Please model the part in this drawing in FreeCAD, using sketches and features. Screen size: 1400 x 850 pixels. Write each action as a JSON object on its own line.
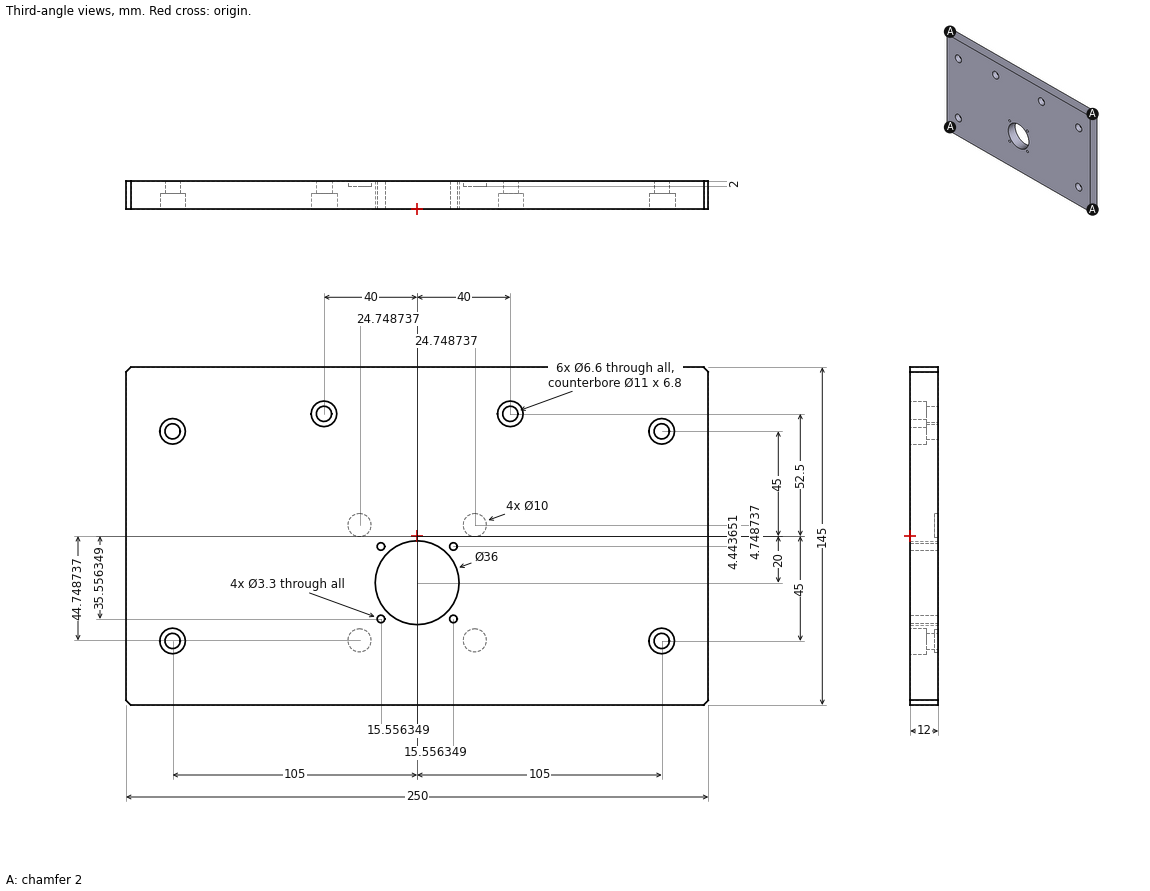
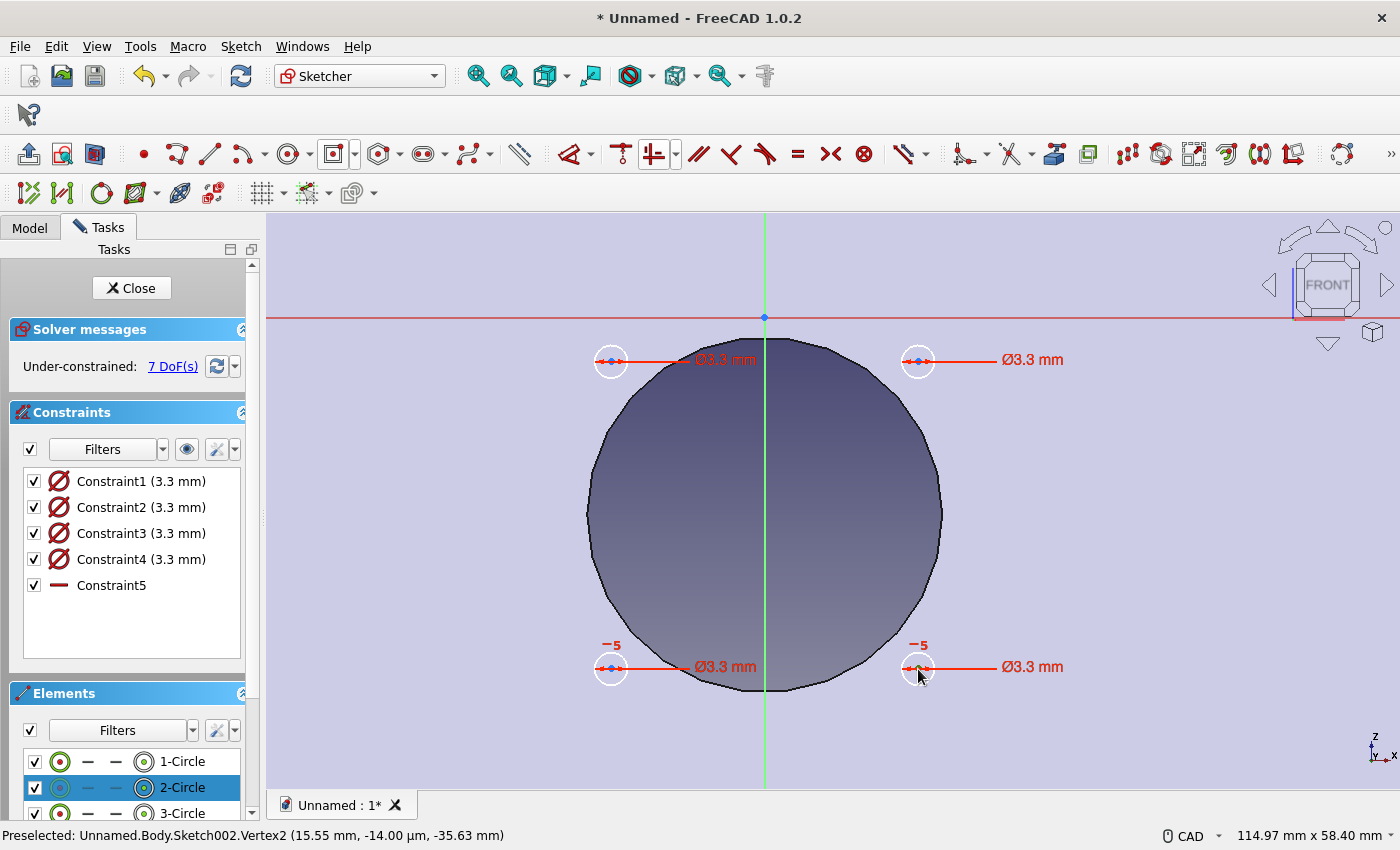
{"action": "left_click", "coordinate": [918, 362]}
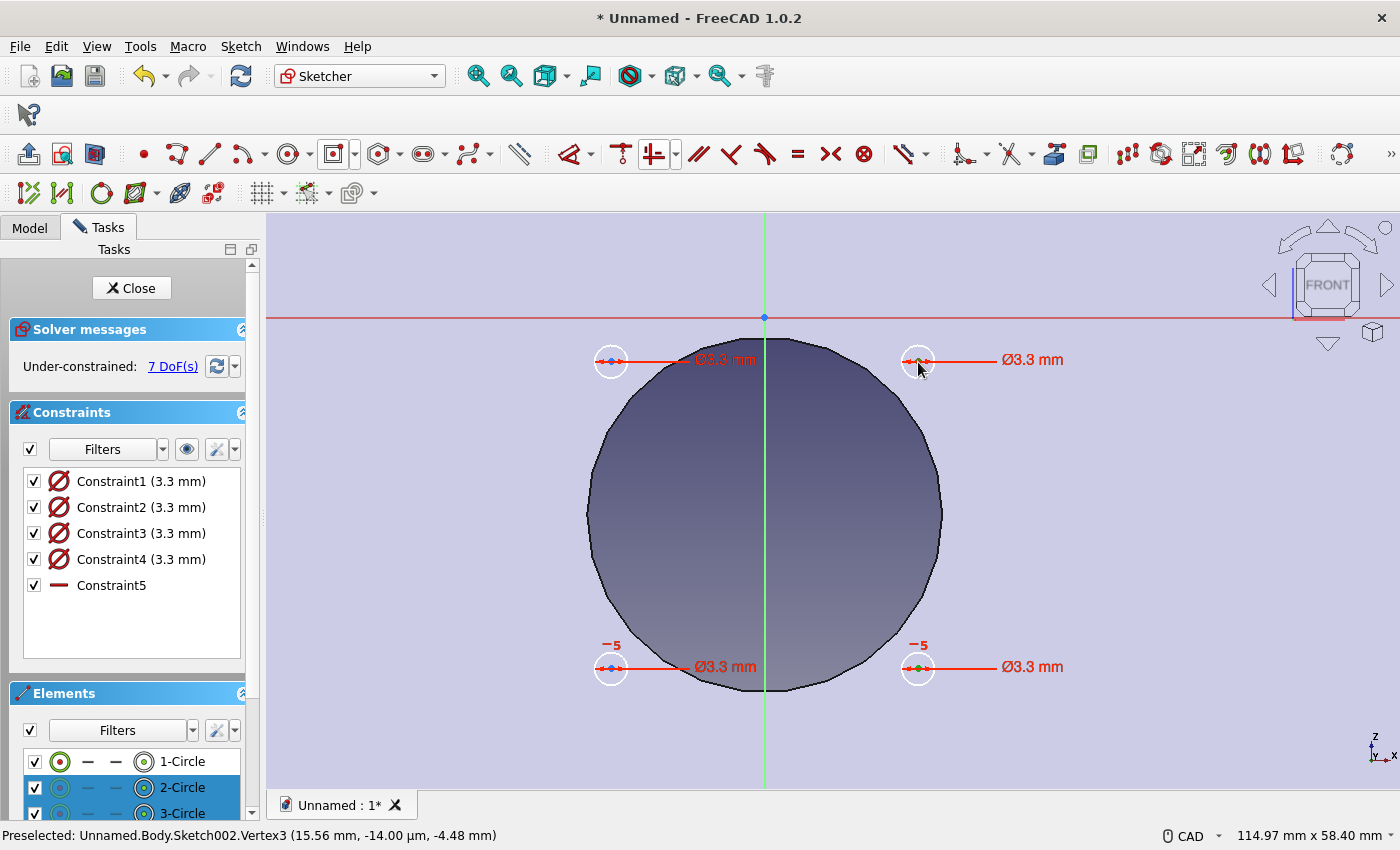
{"action": "key", "text": "v"}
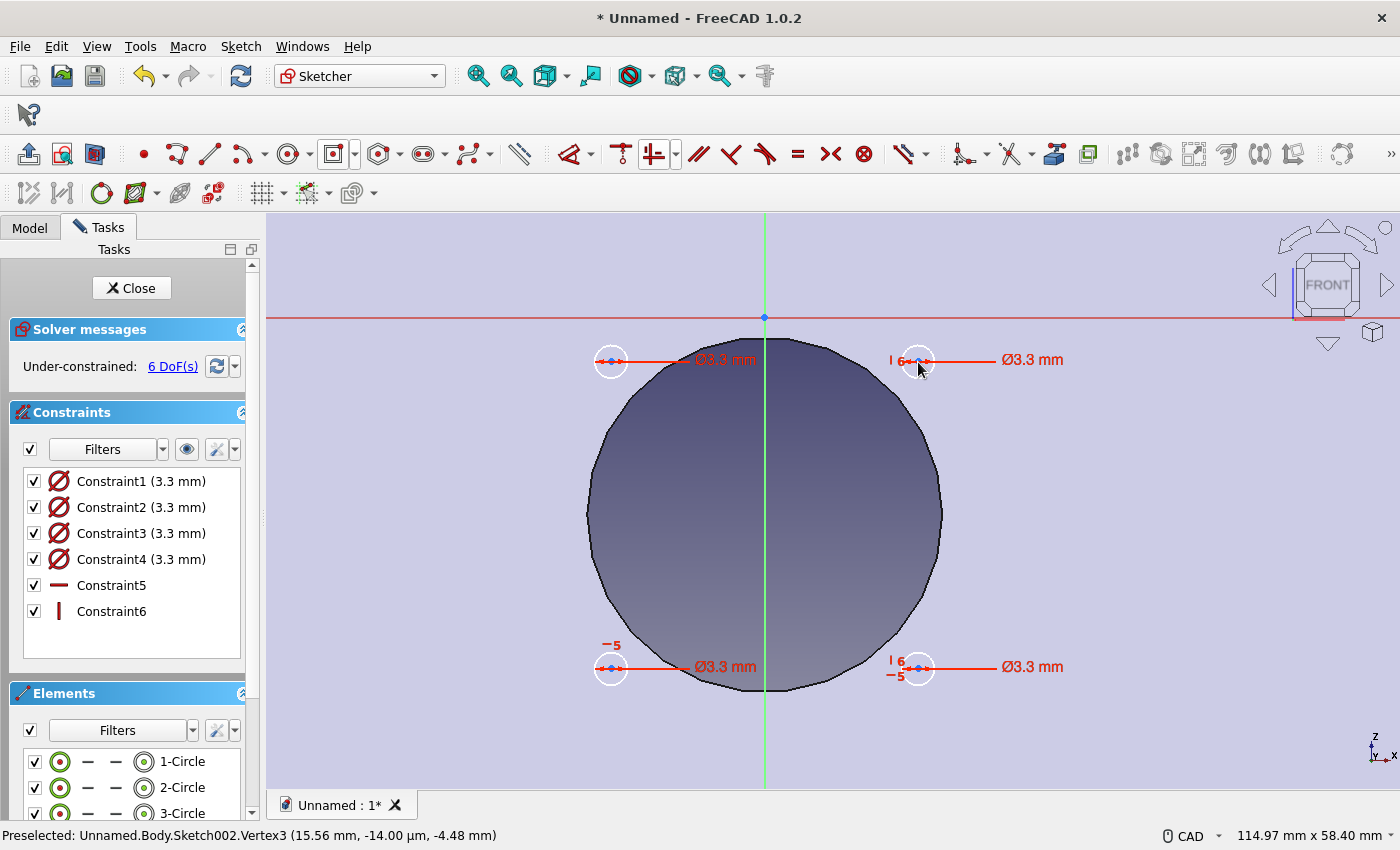
{"action": "left_click", "coordinate": [611, 669]}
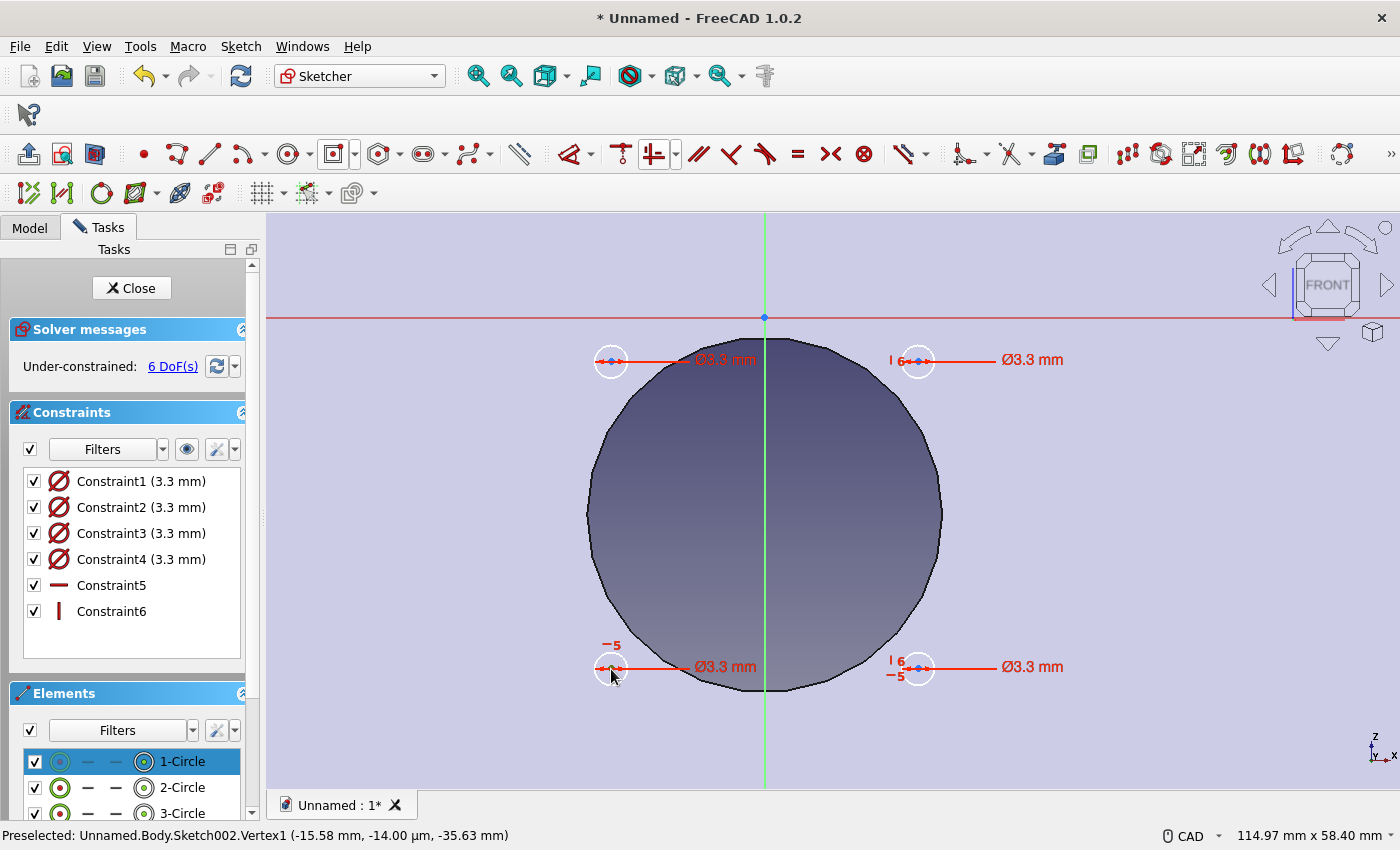
{"action": "left_click", "coordinate": [611, 362]}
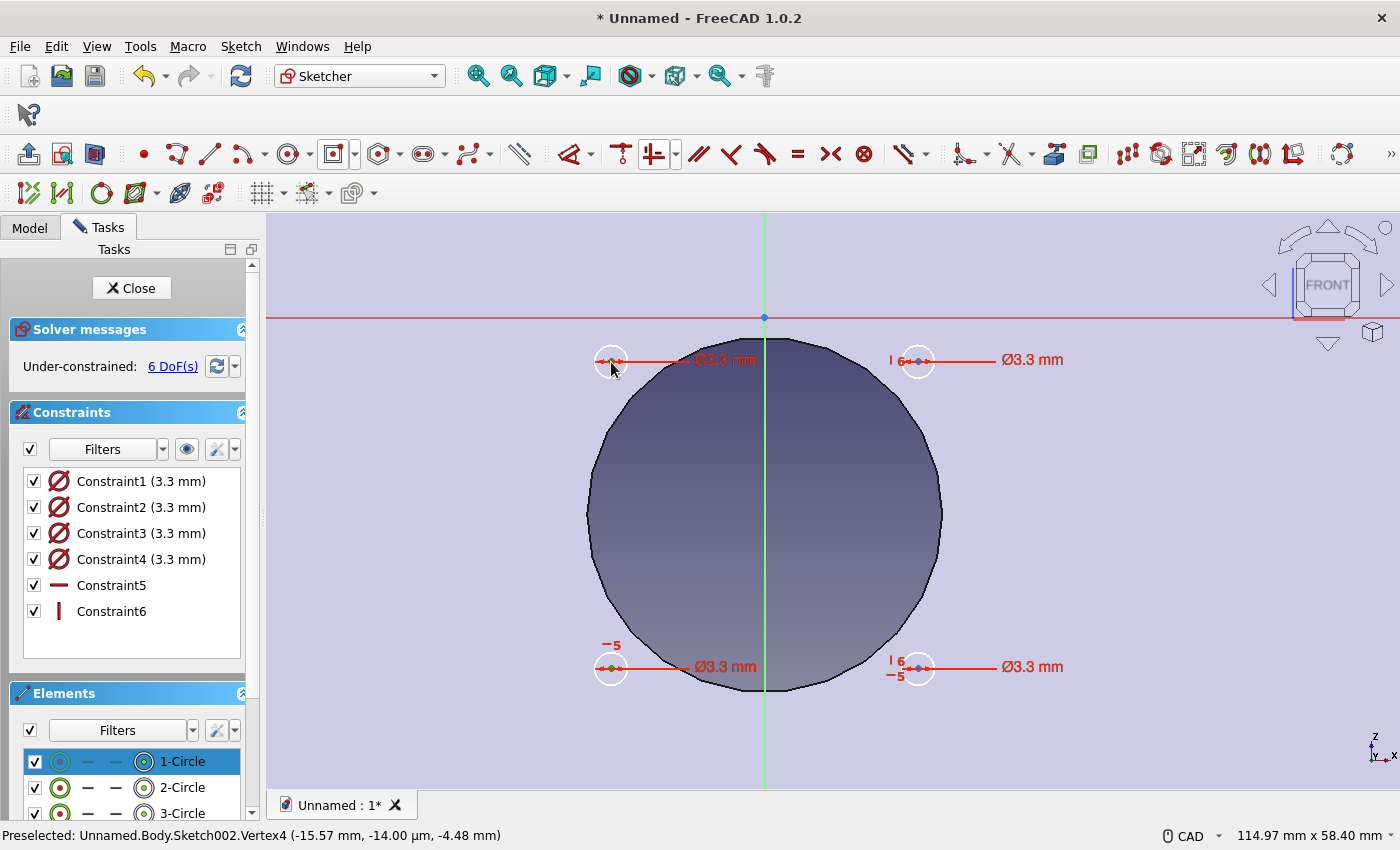
{"action": "left_click", "coordinate": [676, 154]}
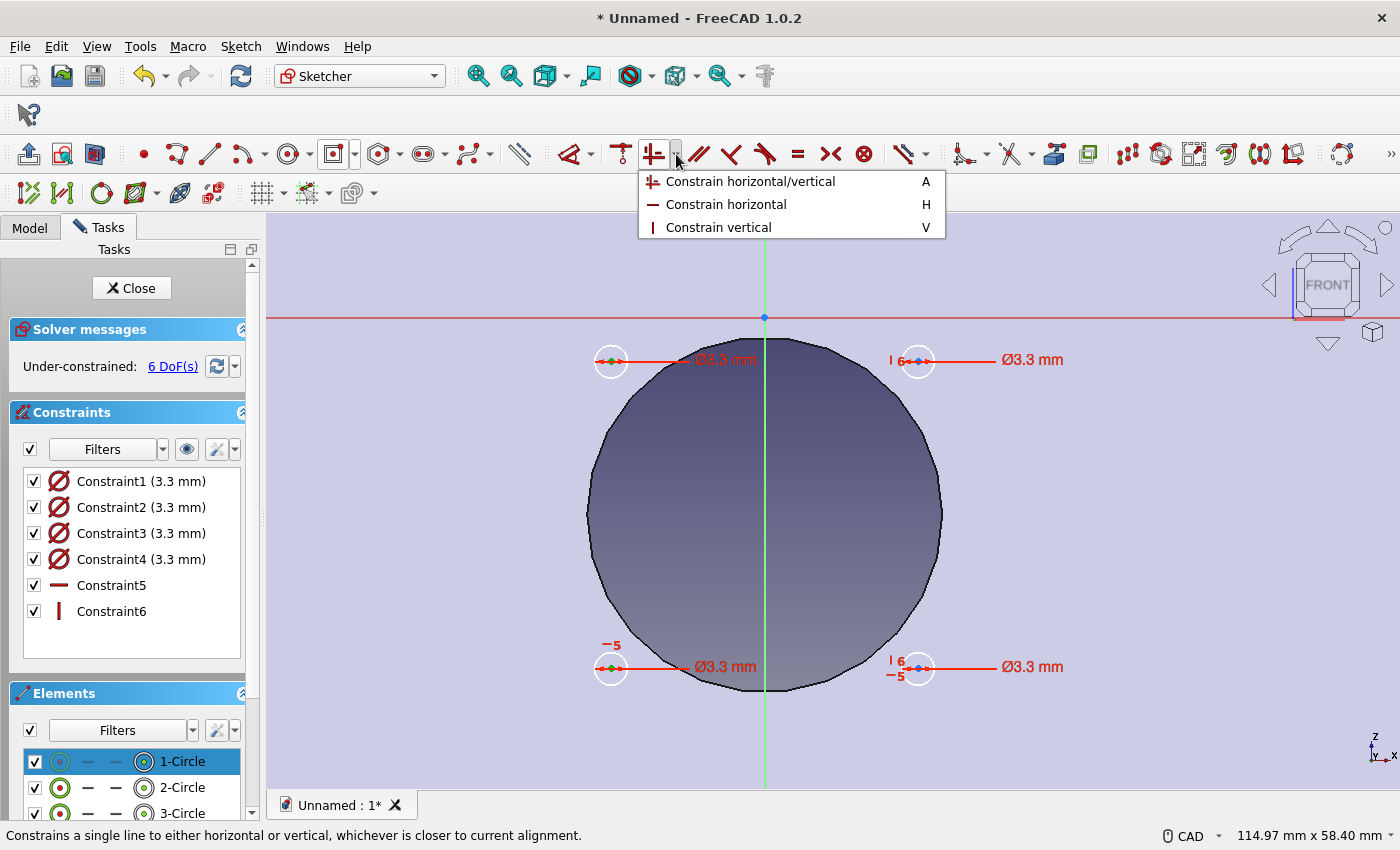
{"action": "left_click", "coordinate": [792, 228]}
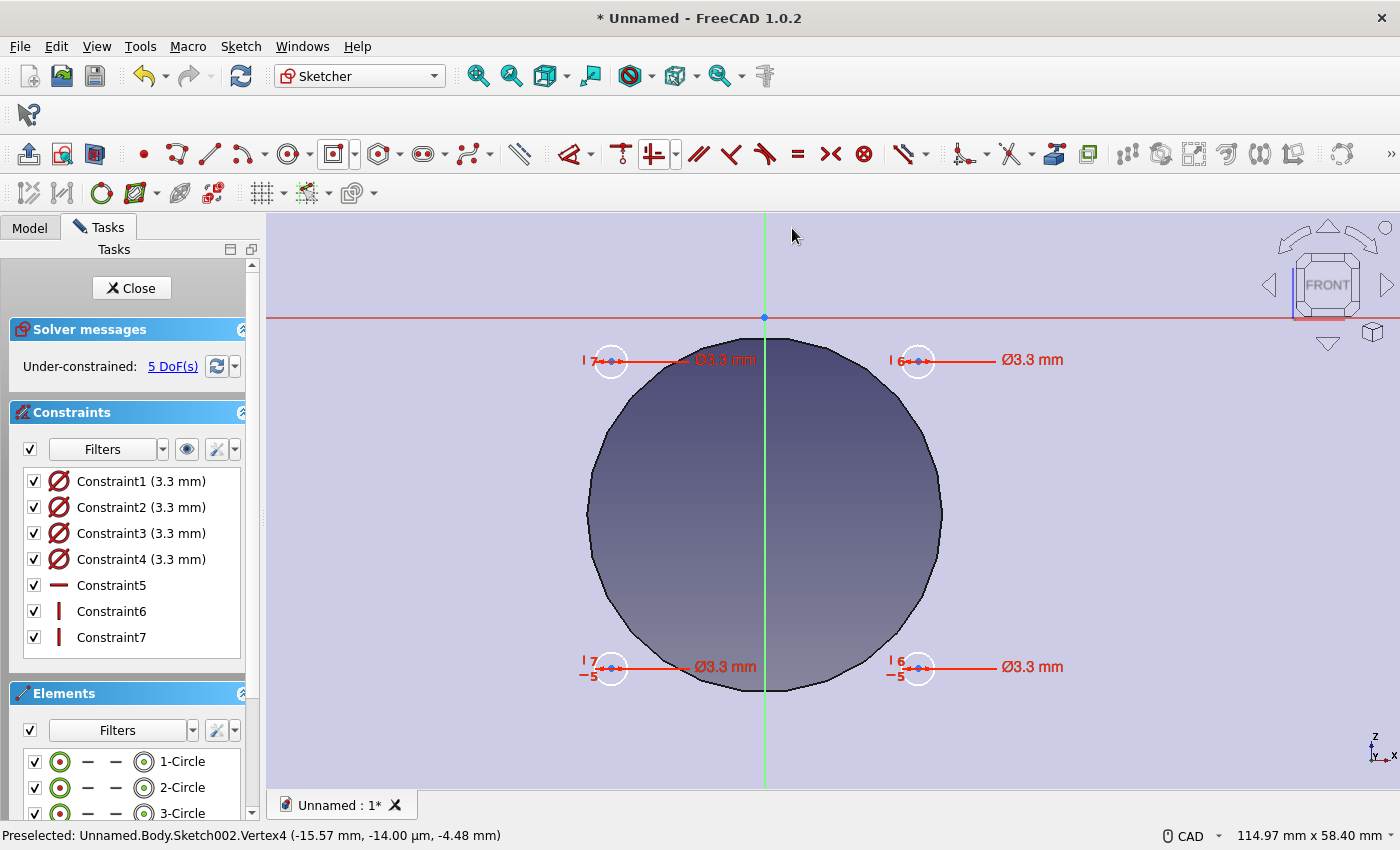
{"action": "left_click", "coordinate": [918, 362]}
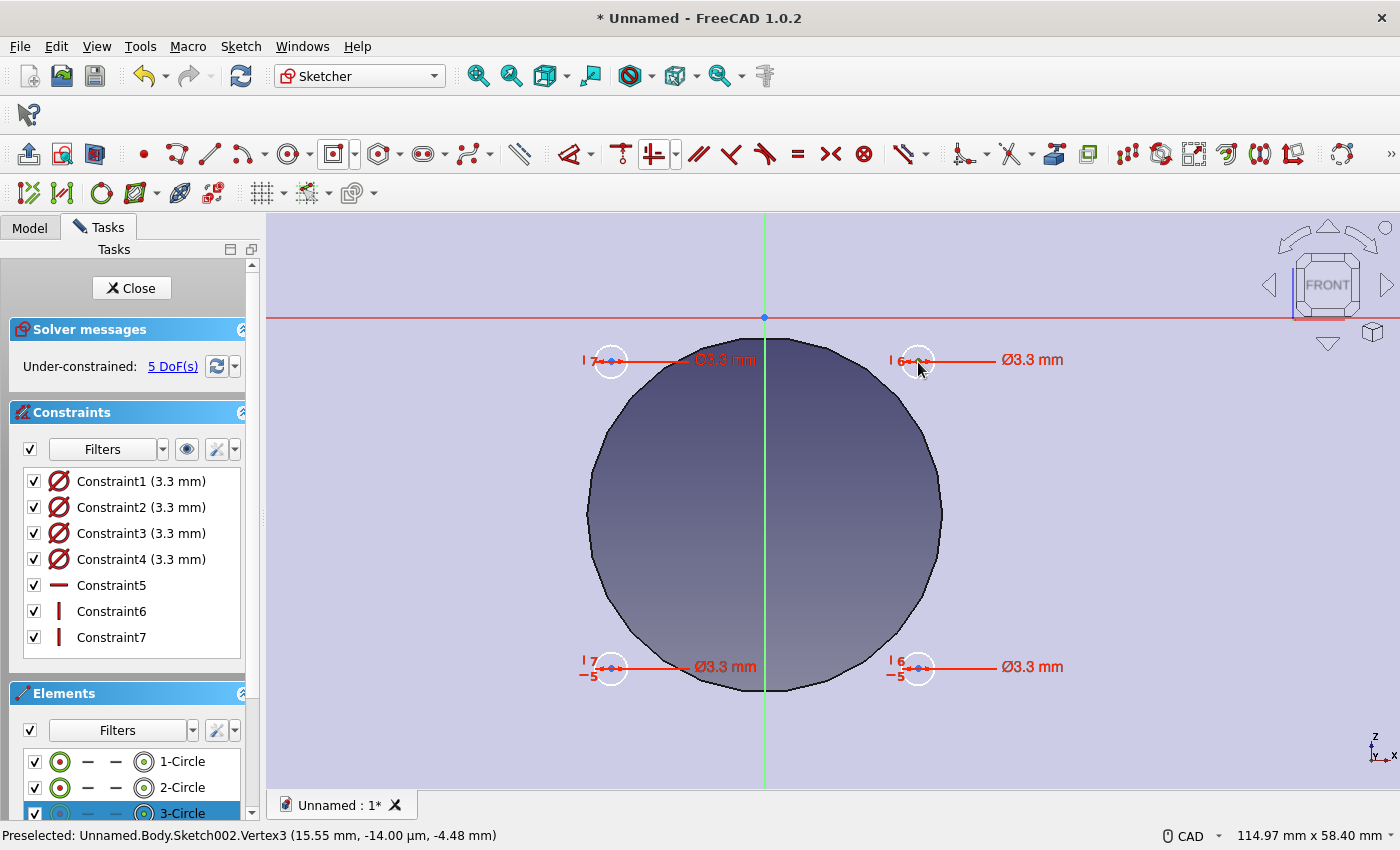
{"action": "left_click", "coordinate": [611, 362]}